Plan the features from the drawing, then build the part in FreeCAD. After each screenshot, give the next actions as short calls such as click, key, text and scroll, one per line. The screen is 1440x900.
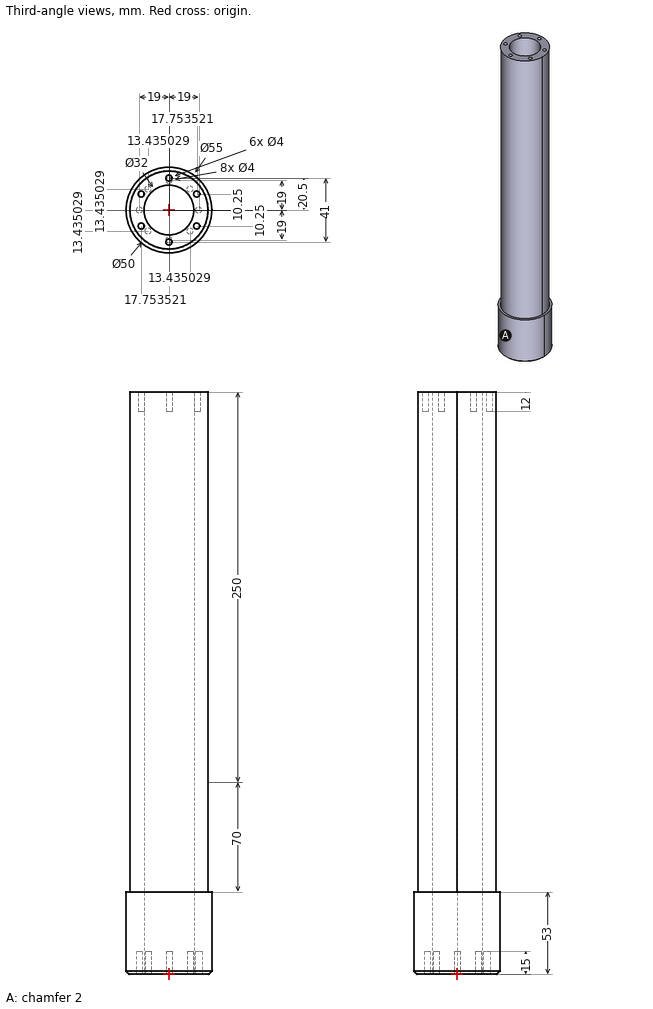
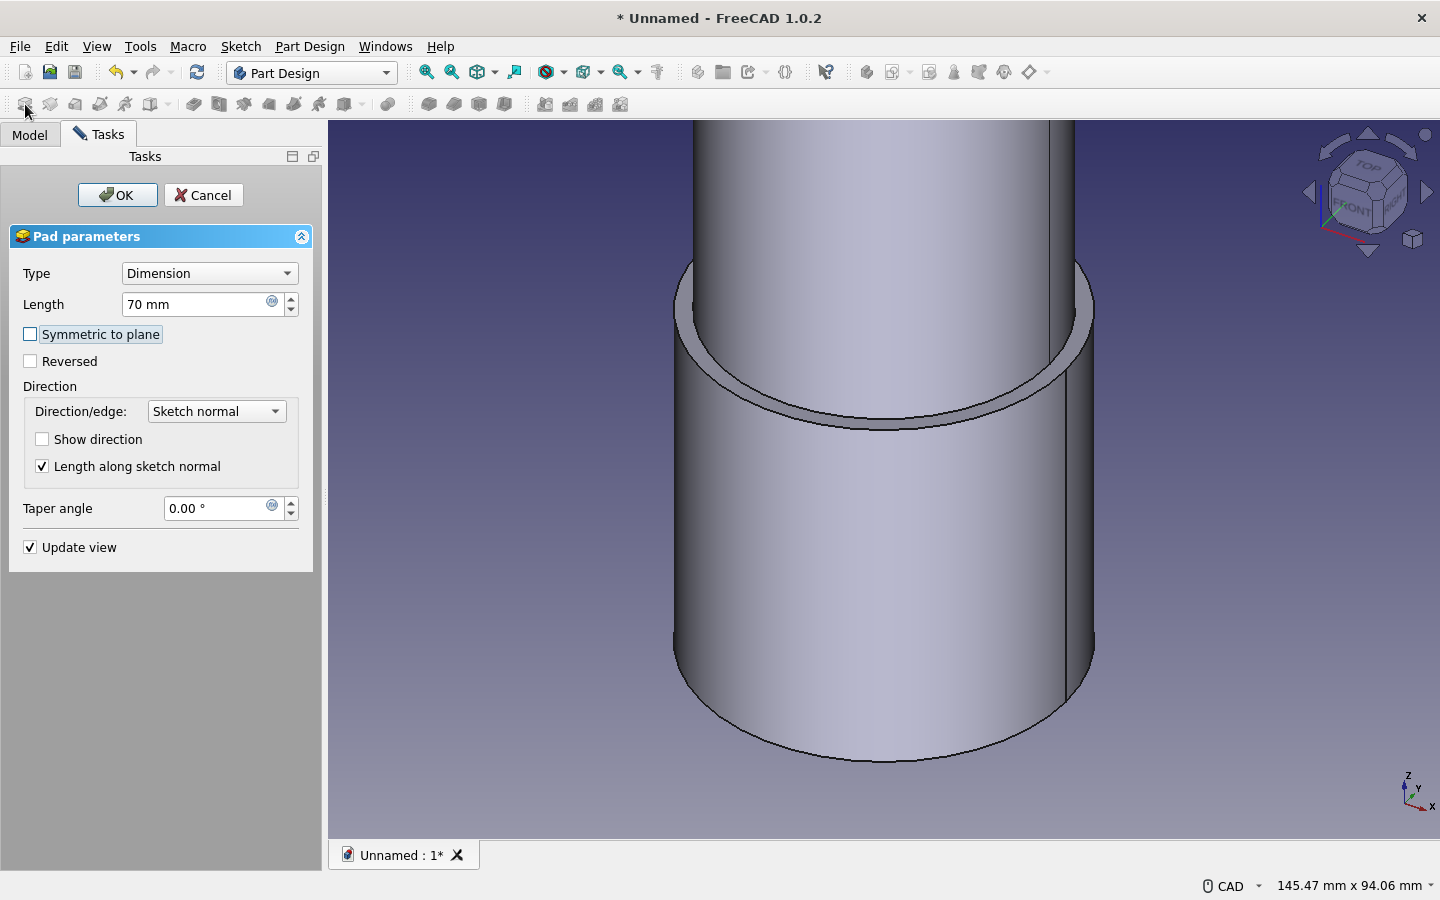
click(118, 195)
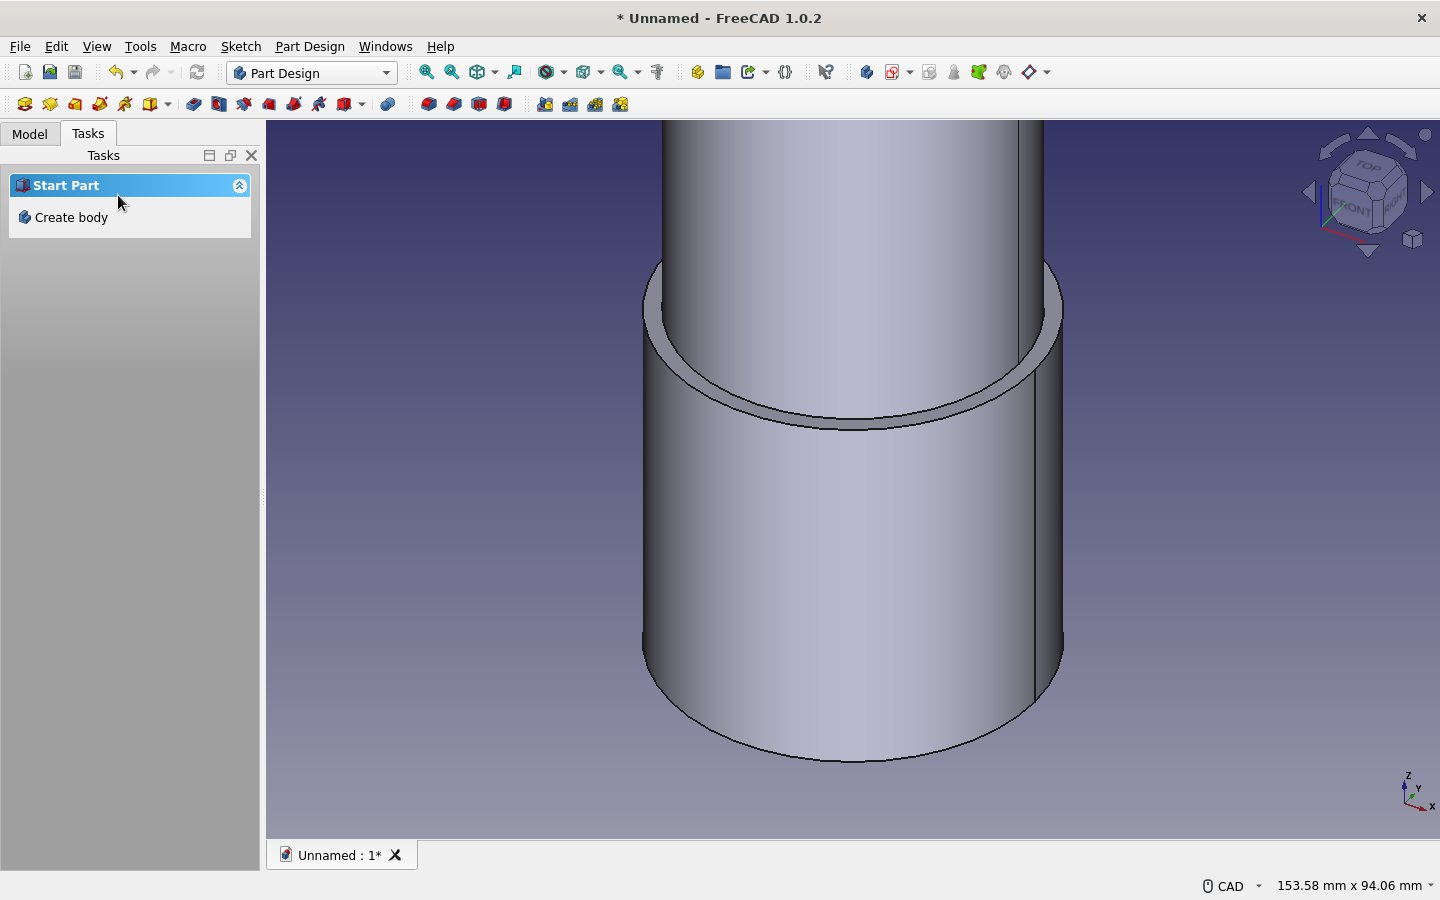
click(427, 72)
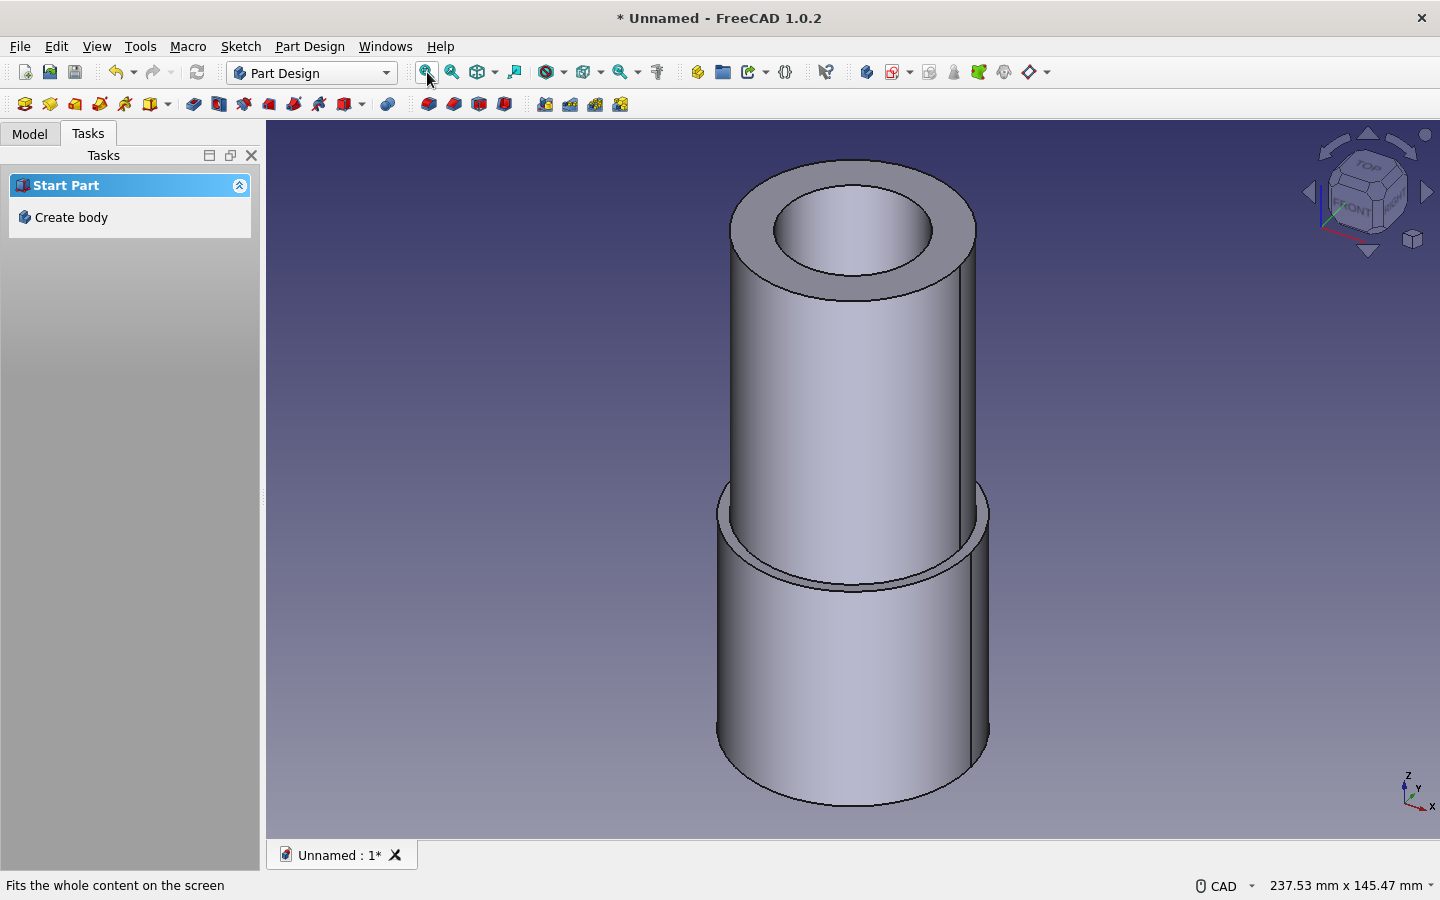
click(892, 72)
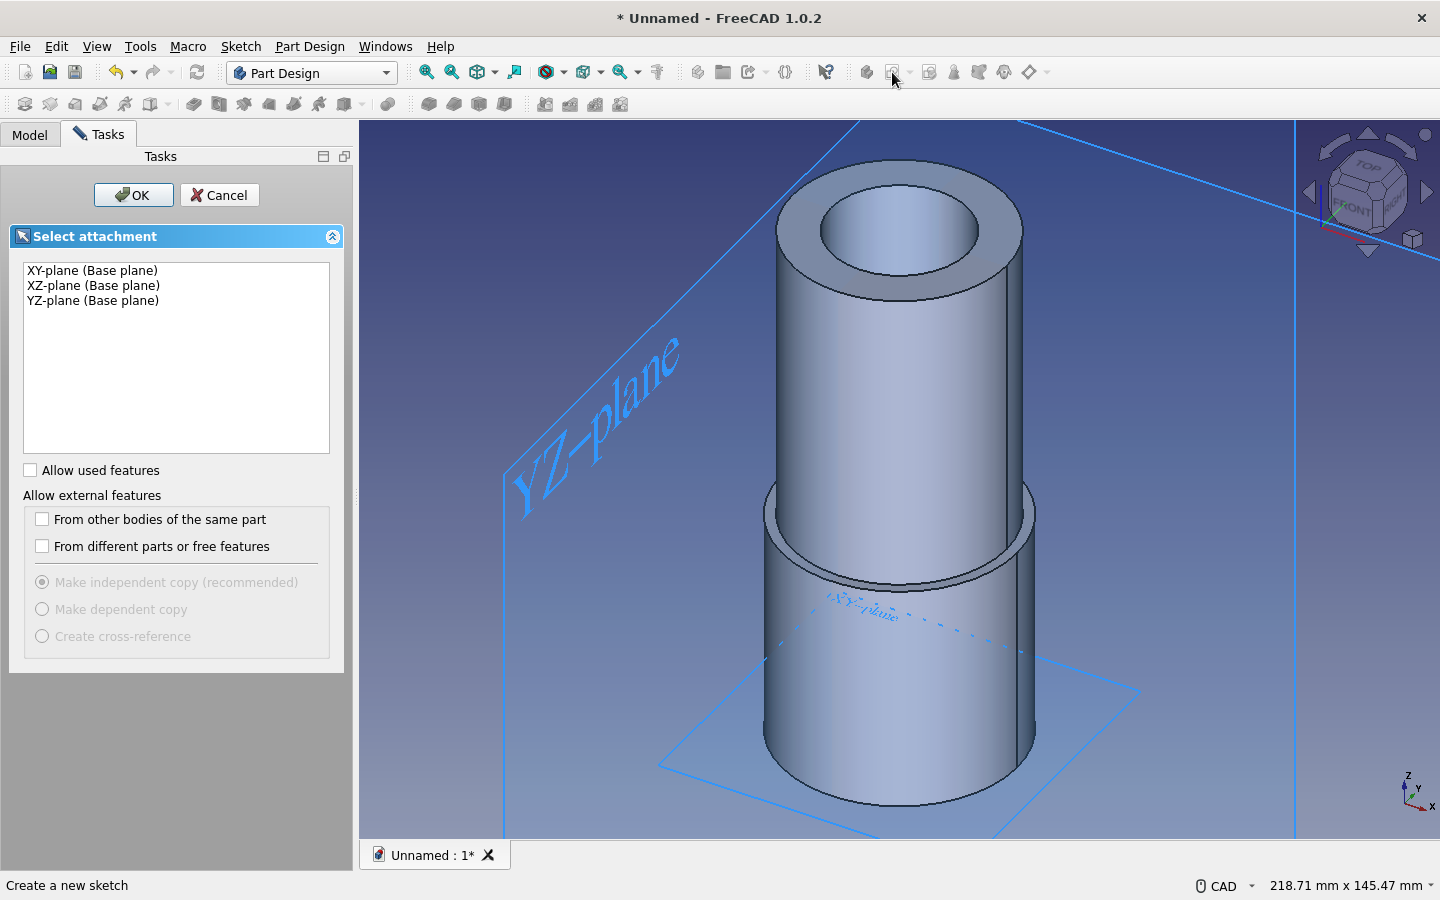
click(84, 270)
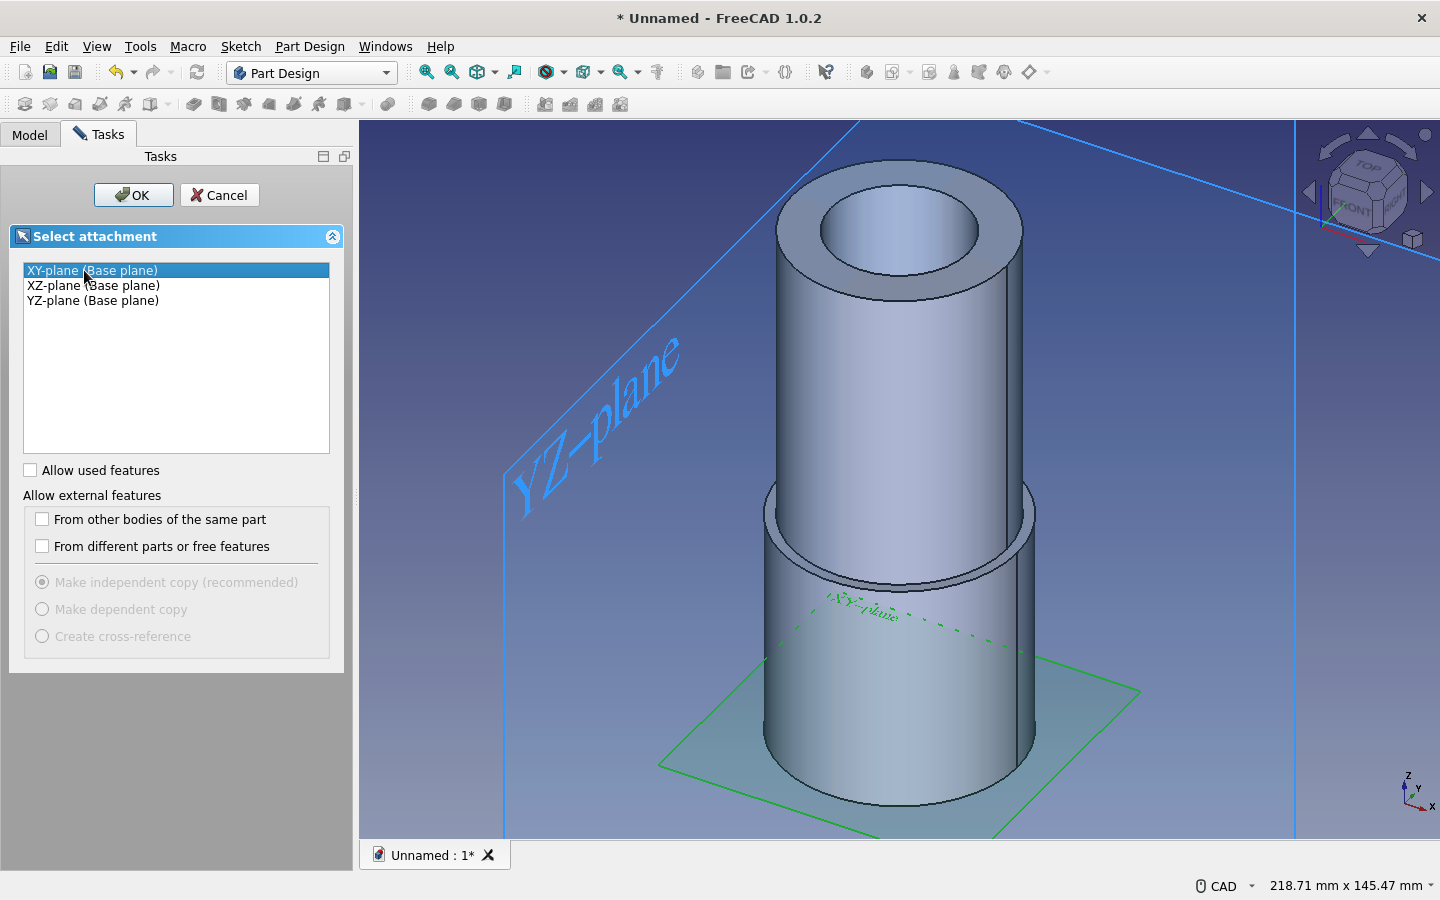
click(134, 195)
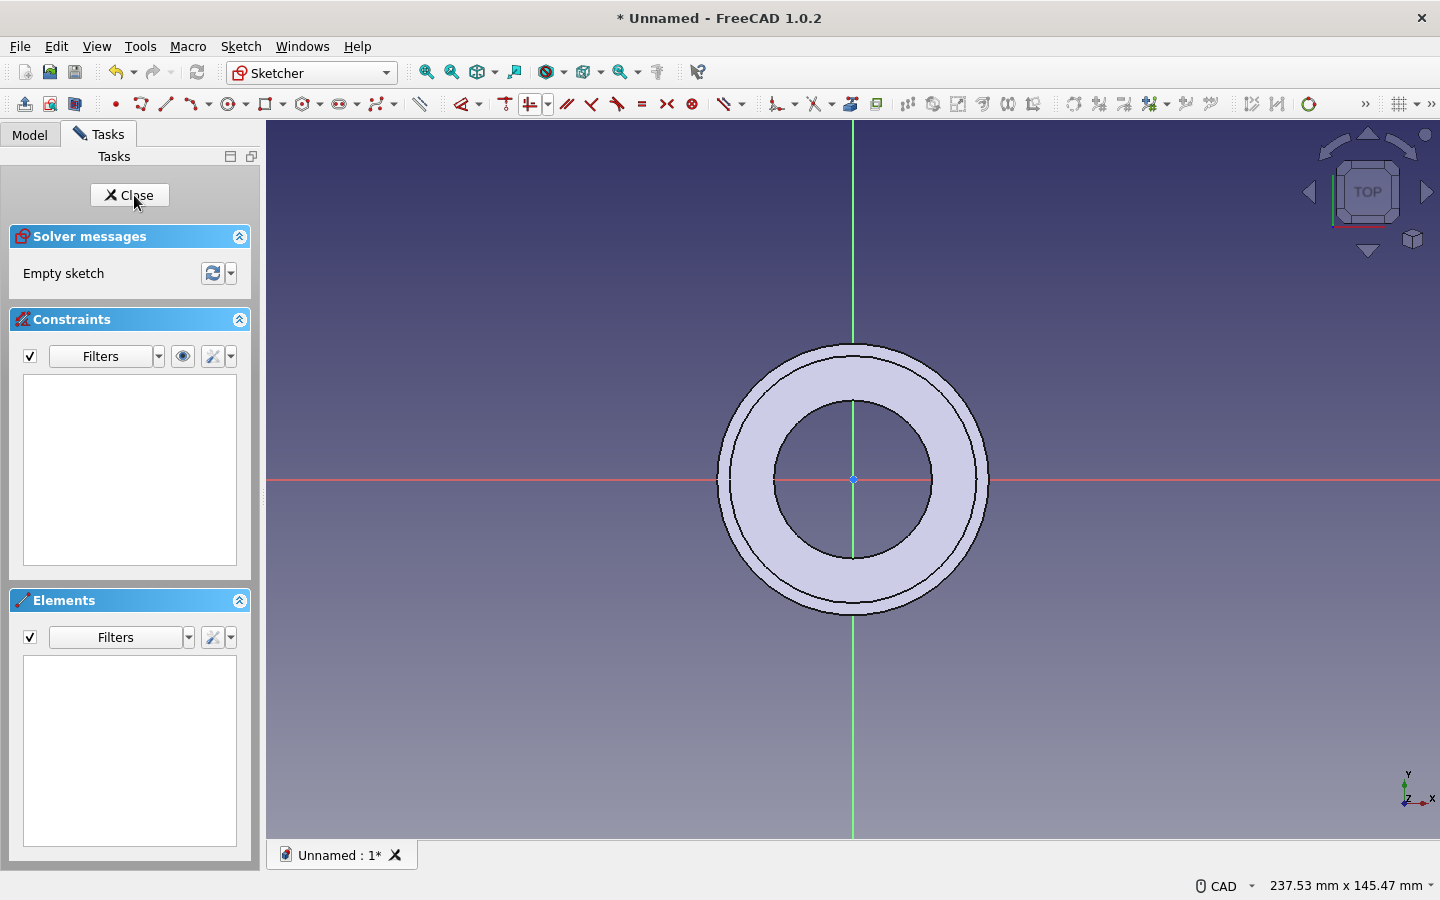
click(75, 104)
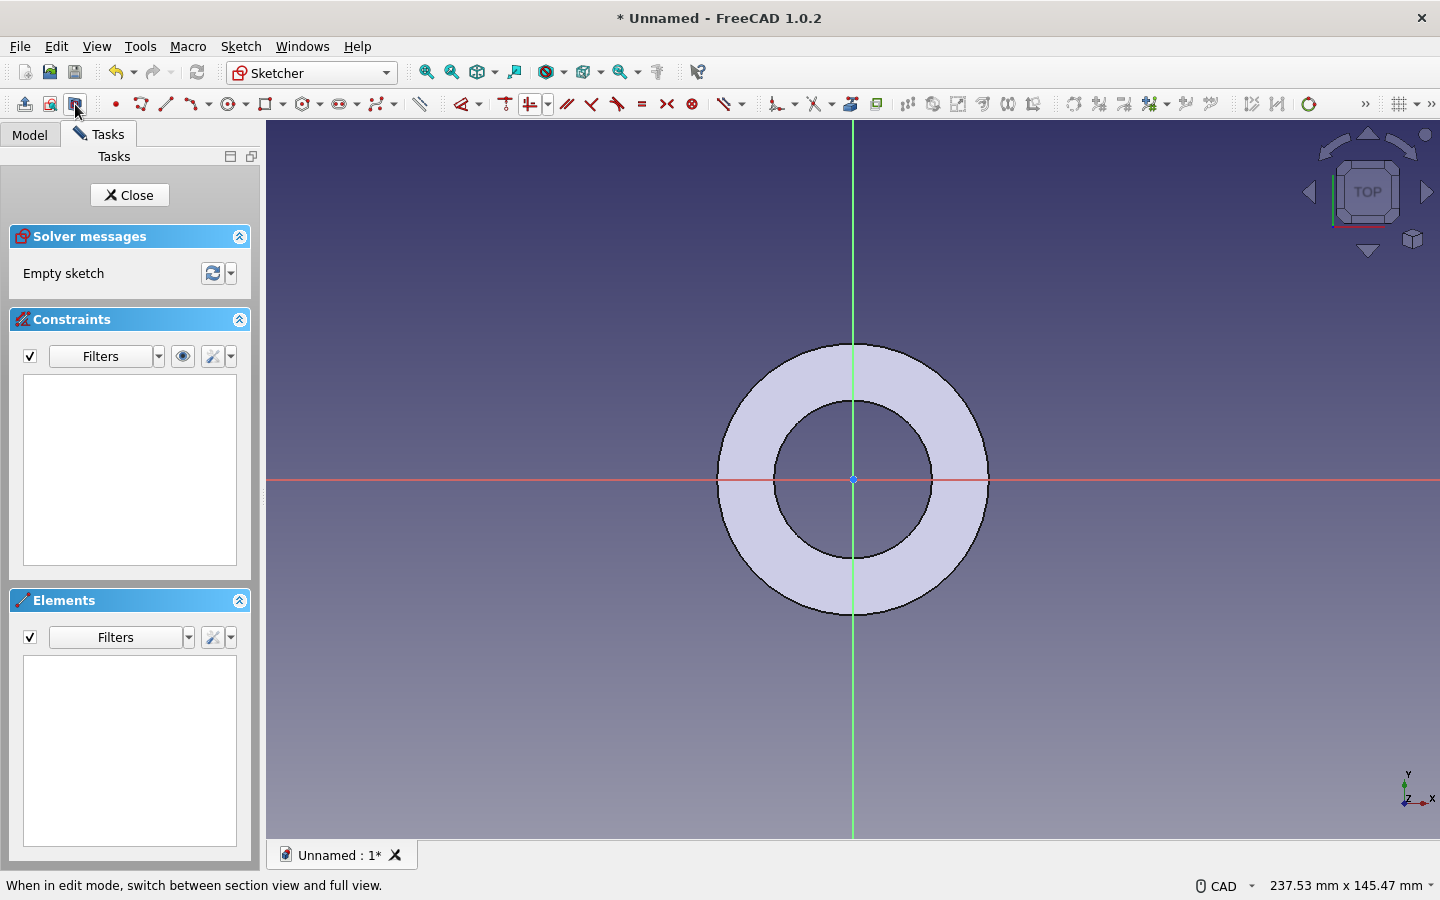
scroll(909, 480, up, 4)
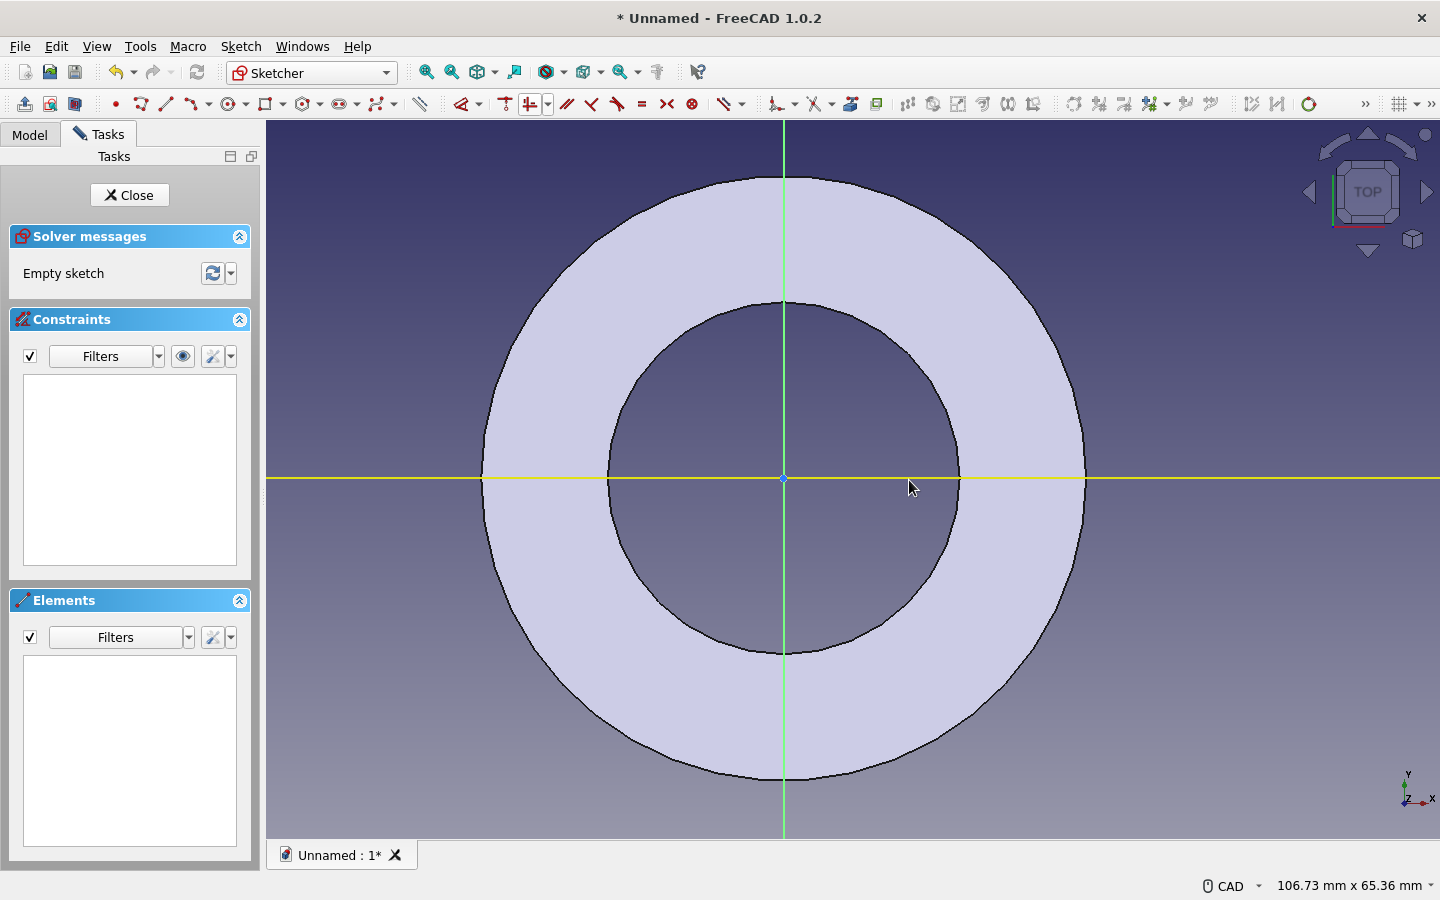
click(228, 104)